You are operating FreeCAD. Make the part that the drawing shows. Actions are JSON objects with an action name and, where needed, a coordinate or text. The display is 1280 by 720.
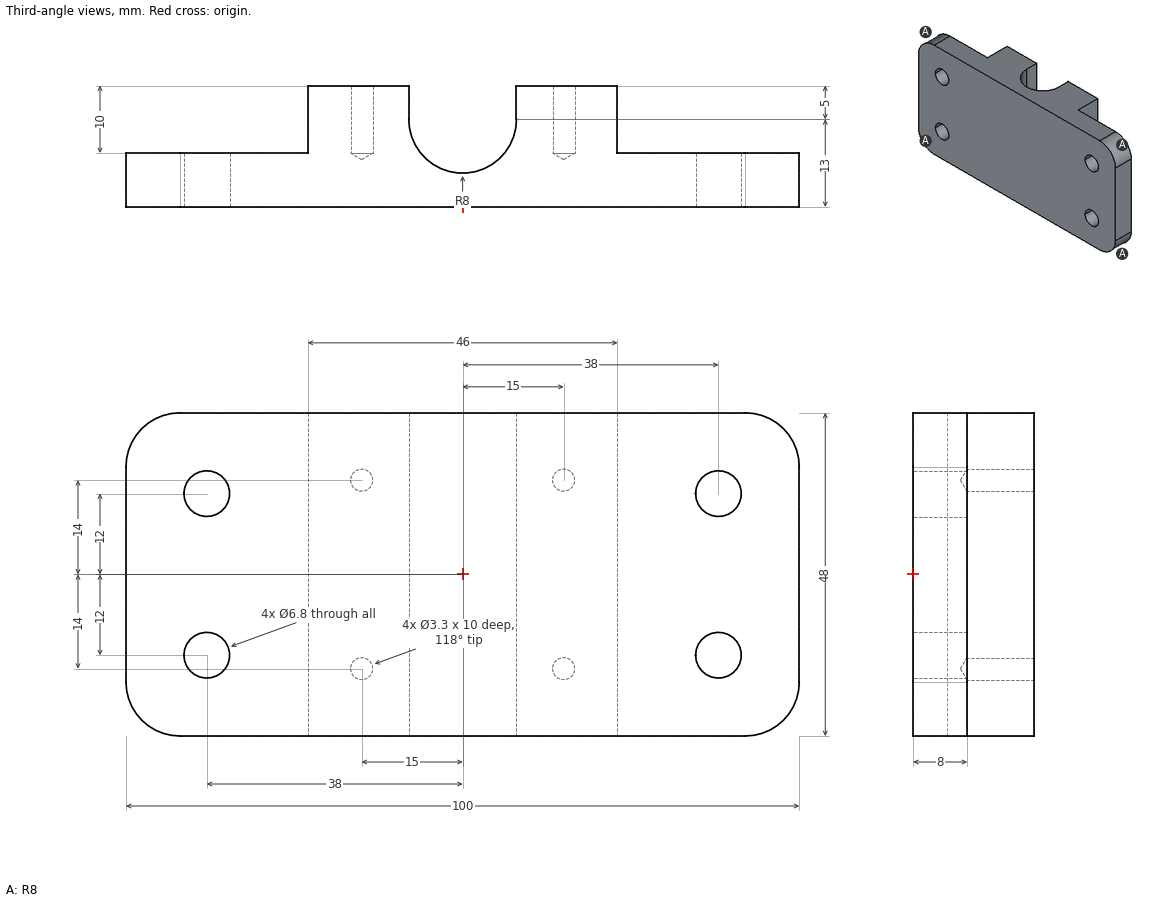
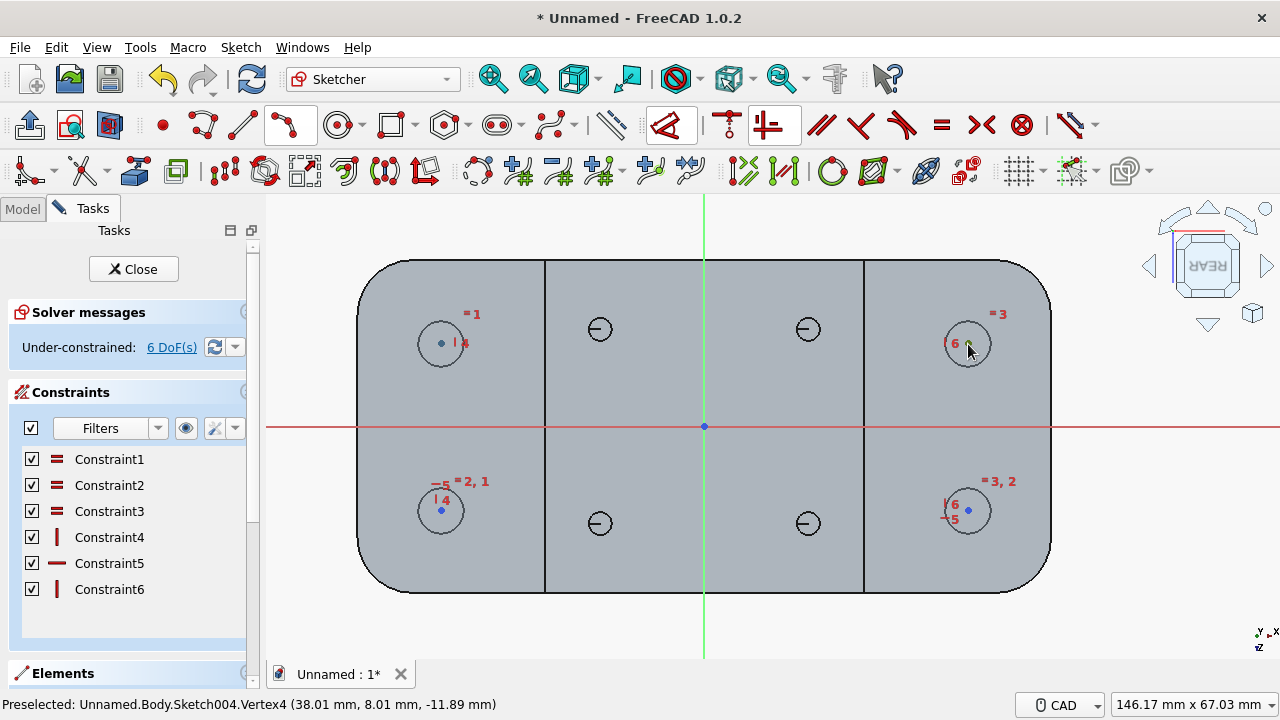
{"action": "left_click", "coordinate": [796, 126]}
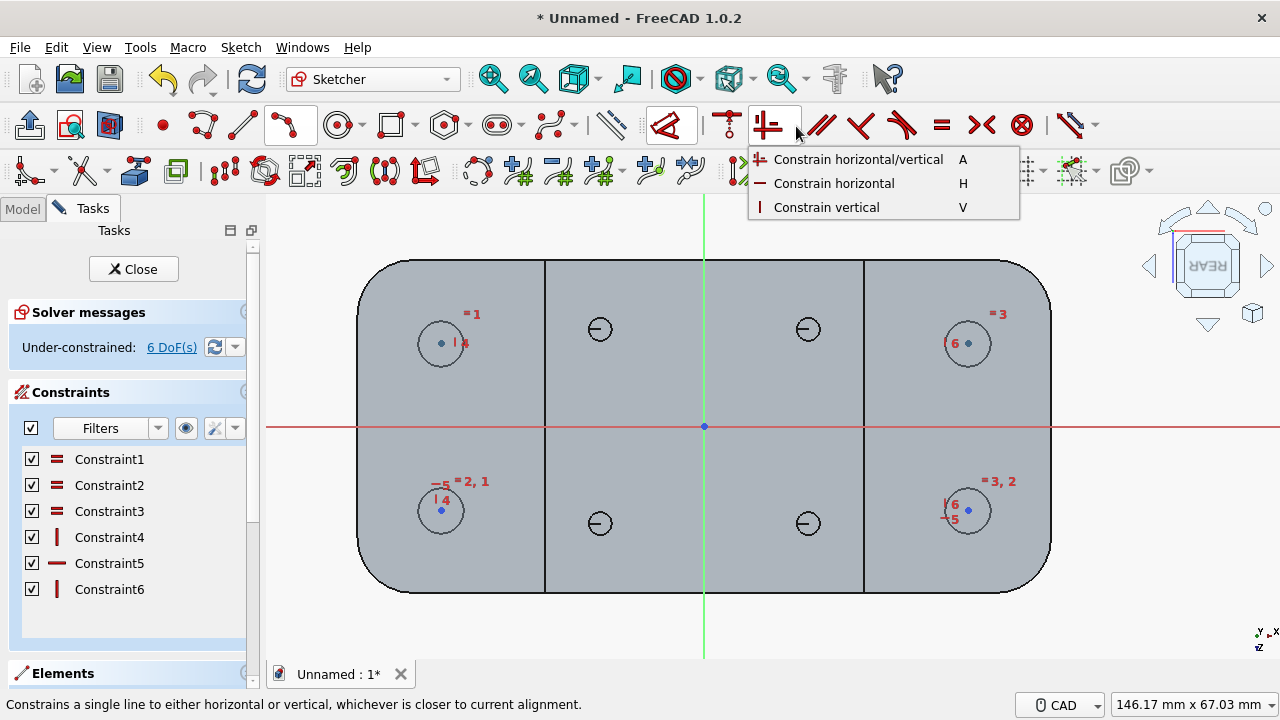
{"action": "left_click", "coordinate": [884, 183]}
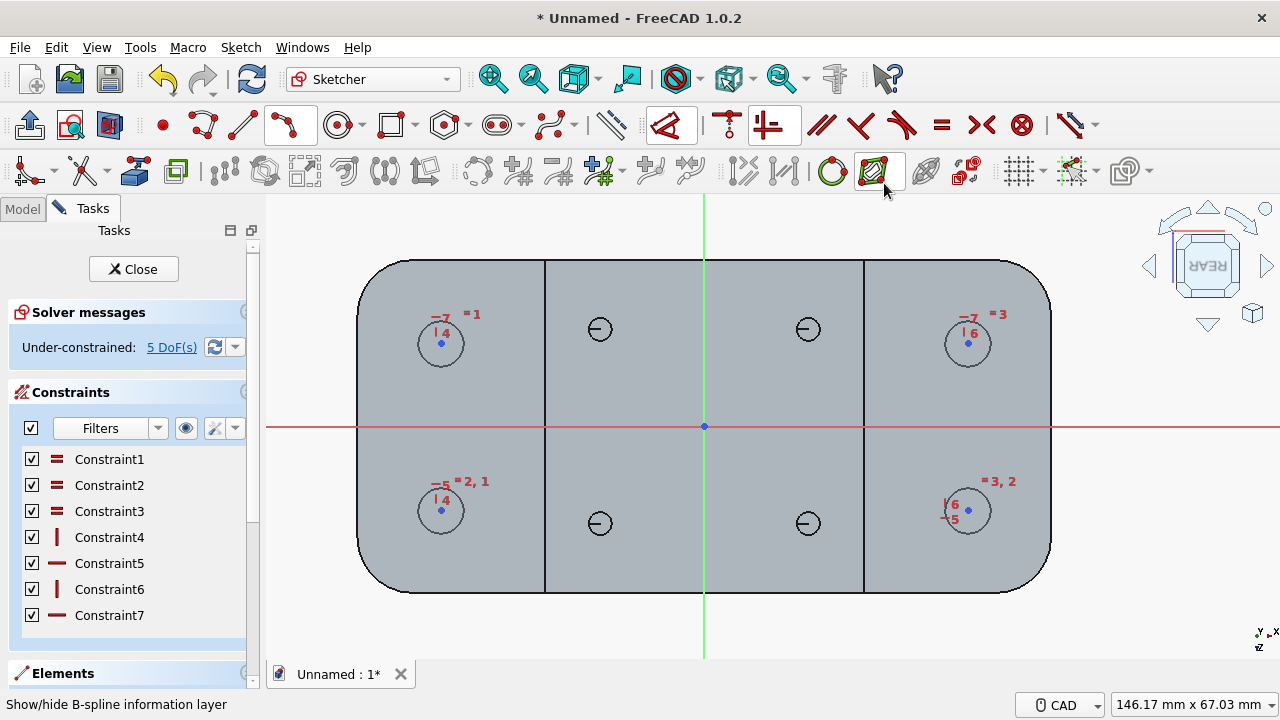
{"action": "left_click", "coordinate": [457, 328]}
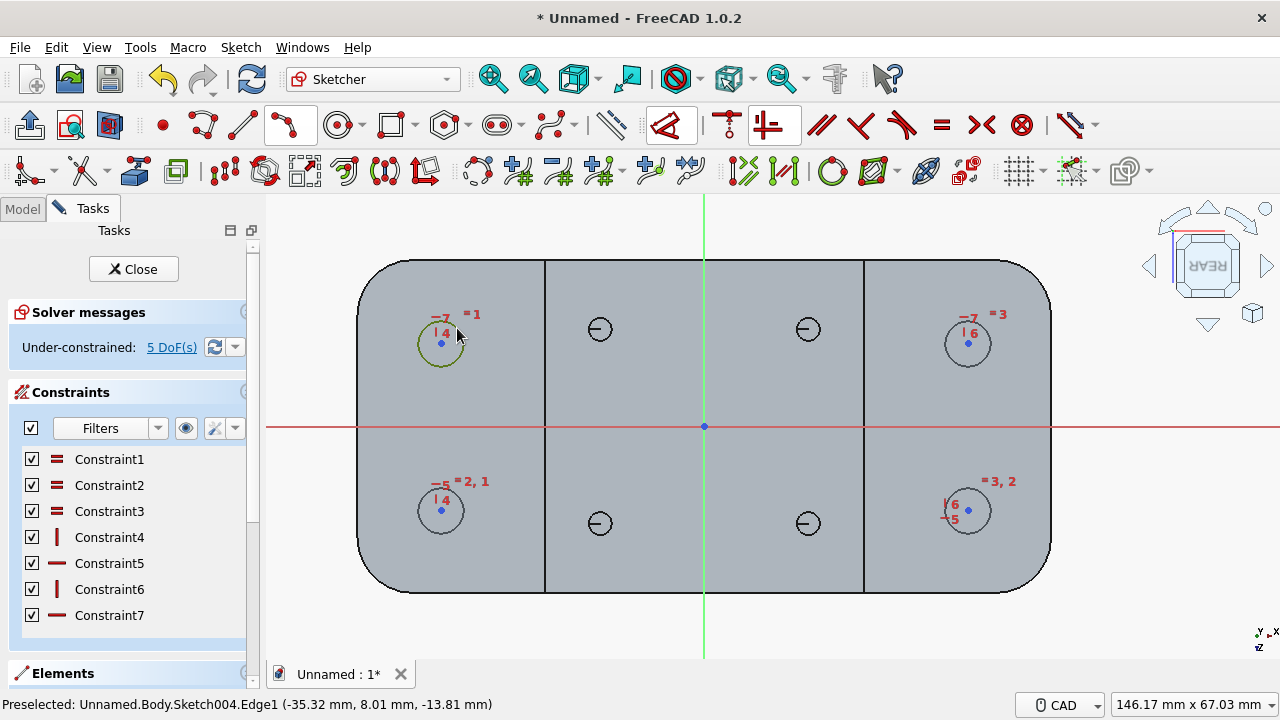
{"action": "left_click", "coordinate": [692, 126]}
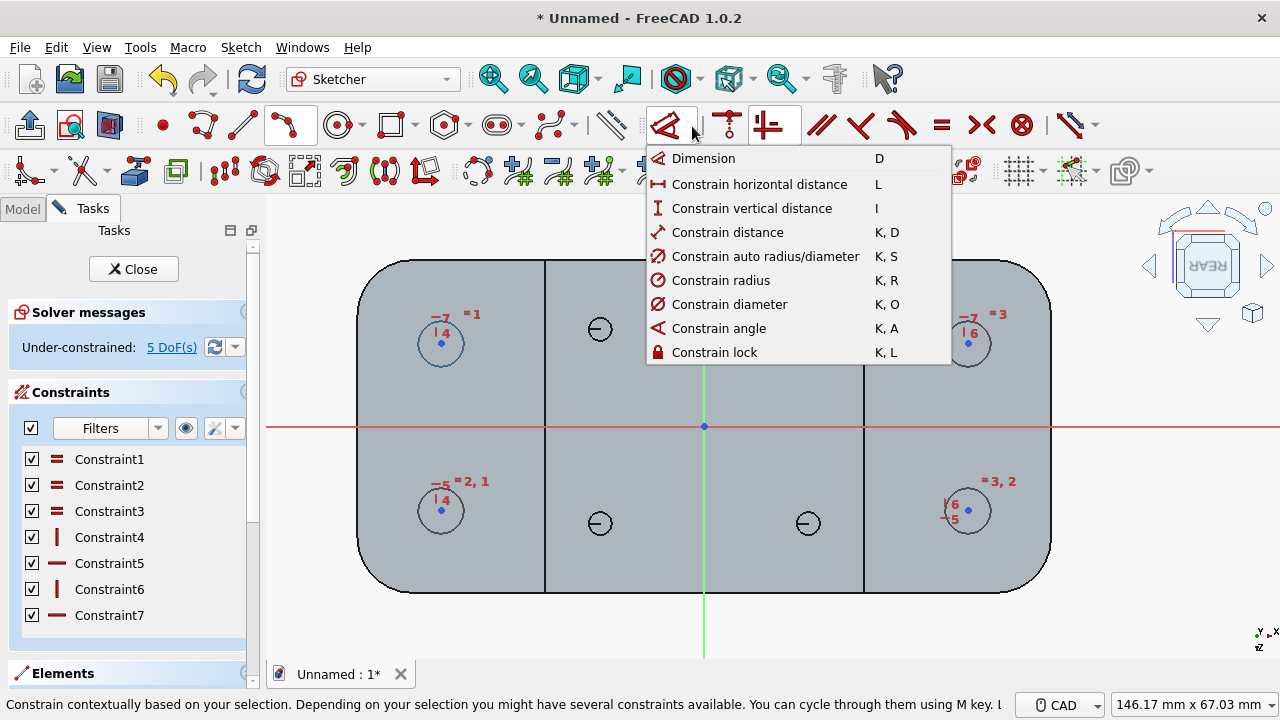
{"action": "left_click", "coordinate": [799, 304]}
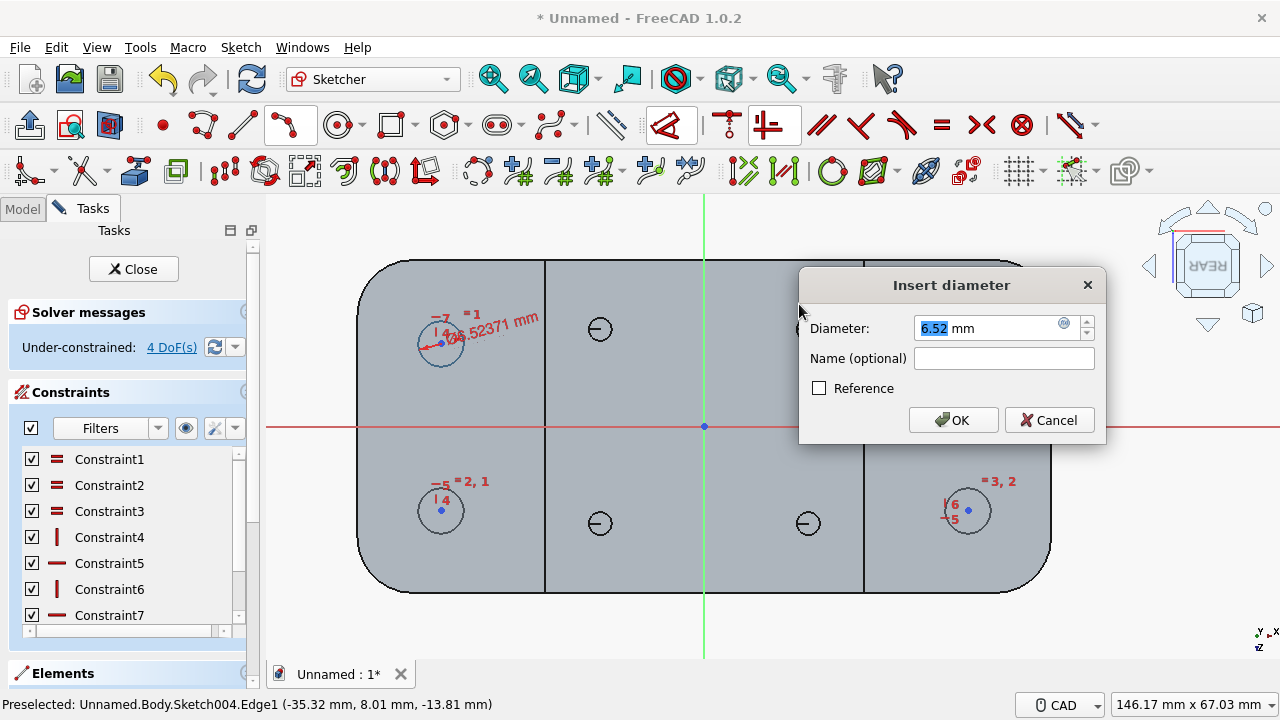
{"action": "type", "text": "6.8"}
{"action": "key", "text": "Return"}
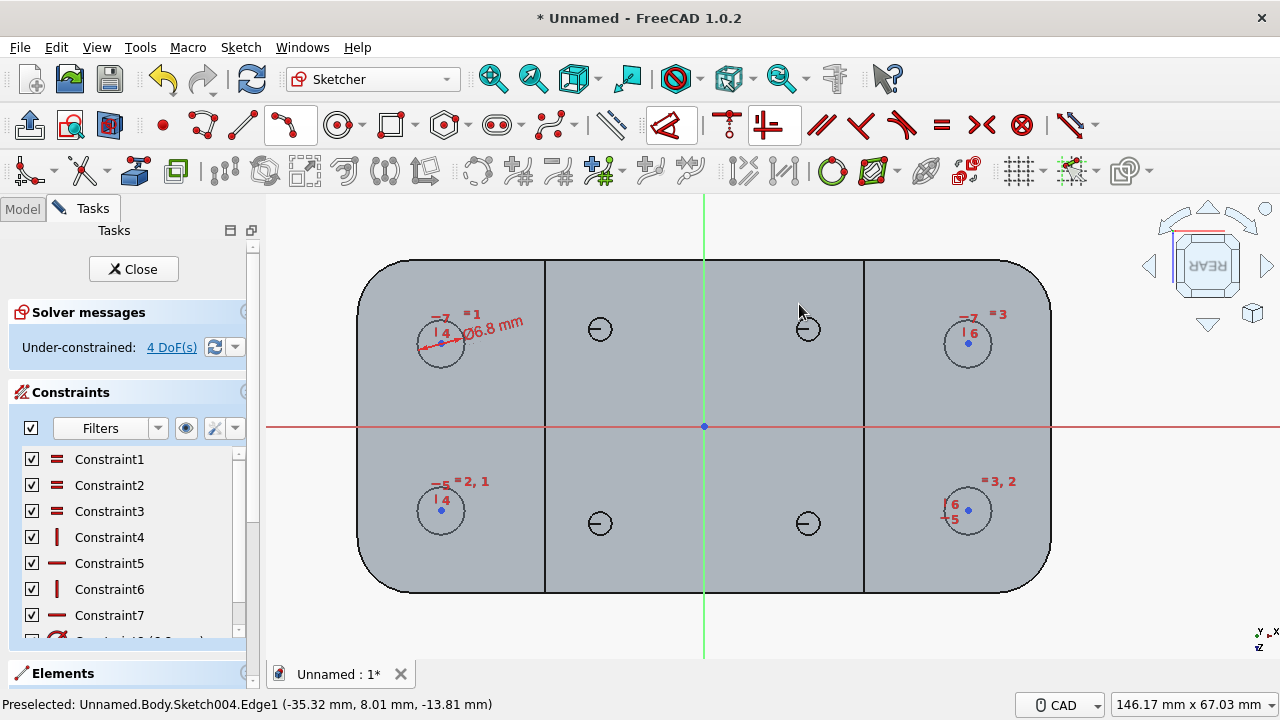
{"action": "left_click", "coordinate": [441, 344]}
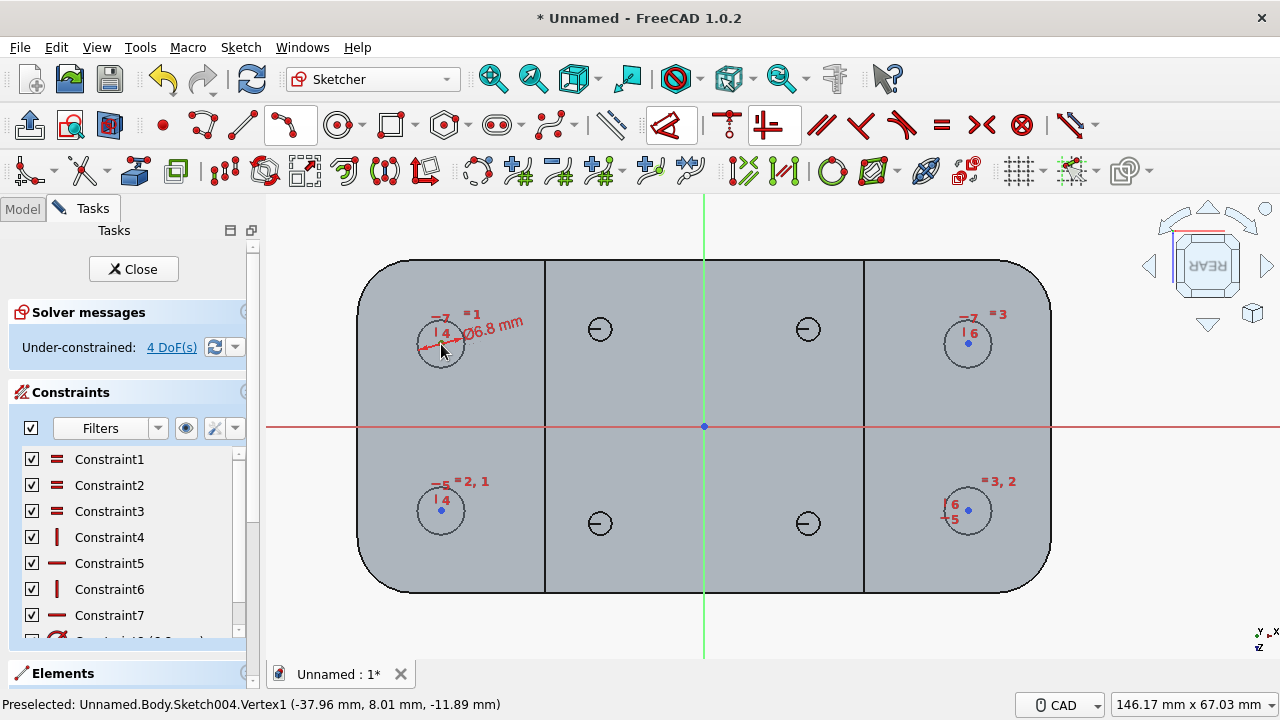
{"action": "left_click", "coordinate": [692, 126]}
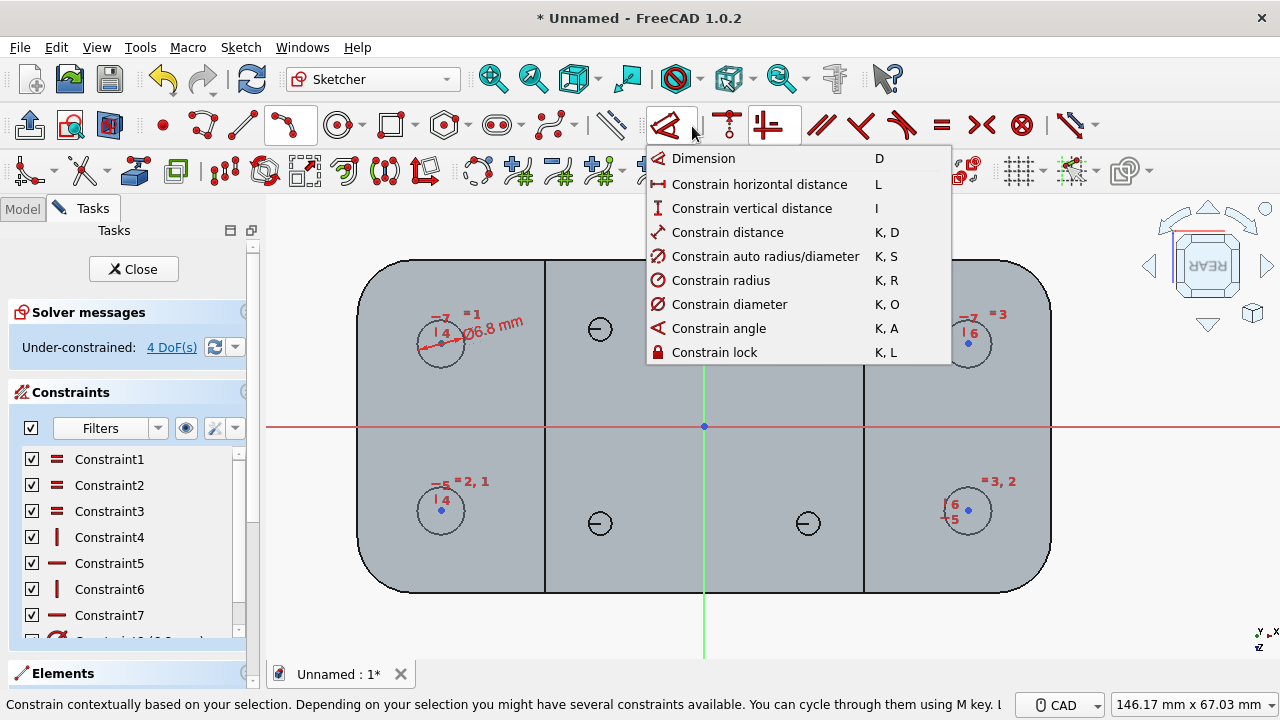
{"action": "left_click", "coordinate": [799, 184]}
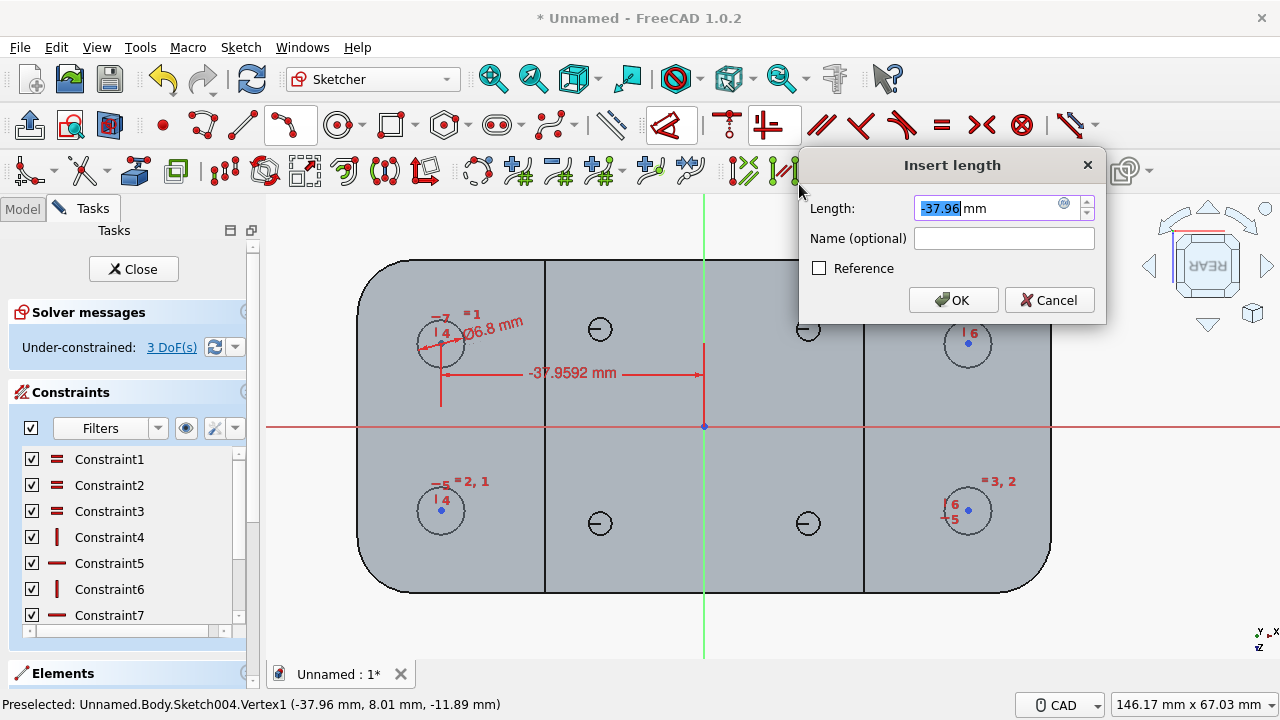
{"action": "type", "text": "-38"}
{"action": "key", "text": "Return"}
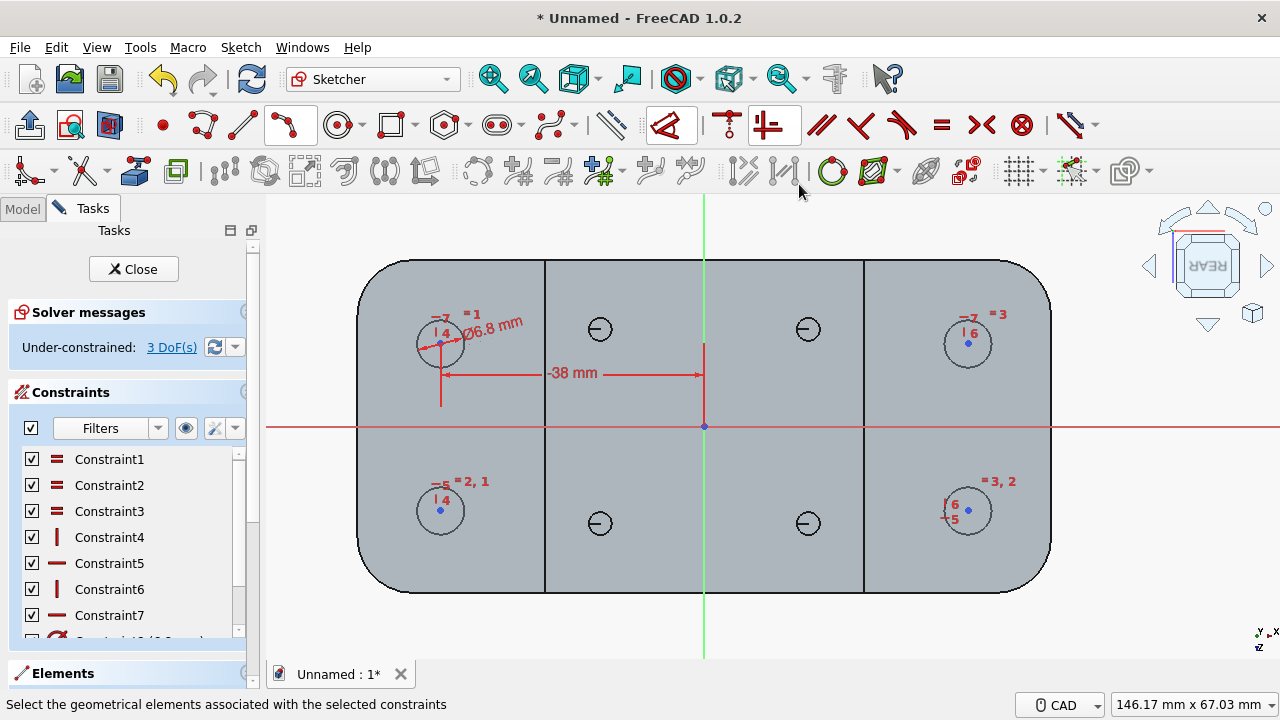
{"action": "left_click", "coordinate": [441, 344]}